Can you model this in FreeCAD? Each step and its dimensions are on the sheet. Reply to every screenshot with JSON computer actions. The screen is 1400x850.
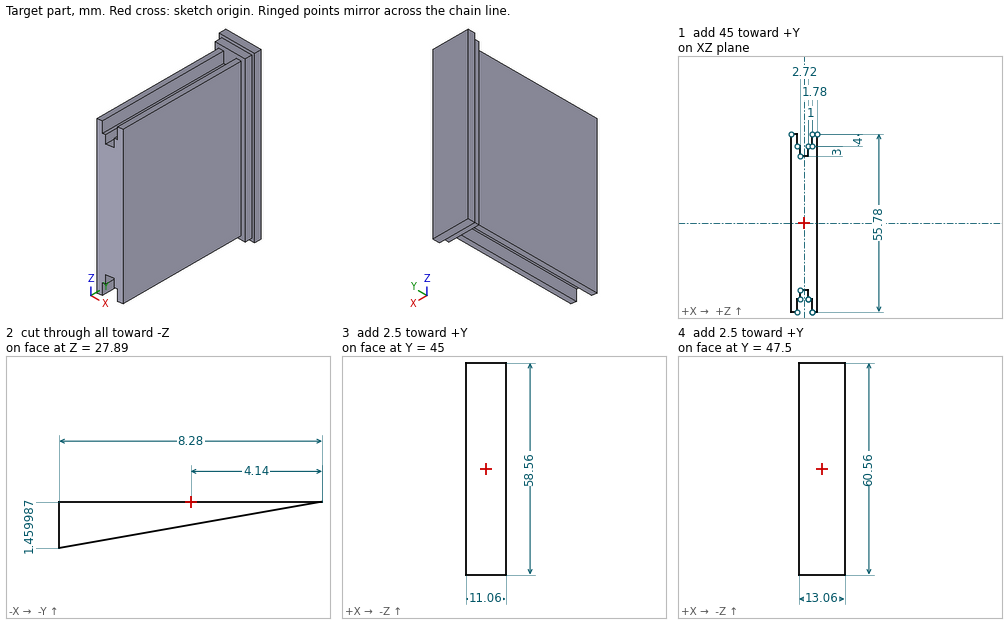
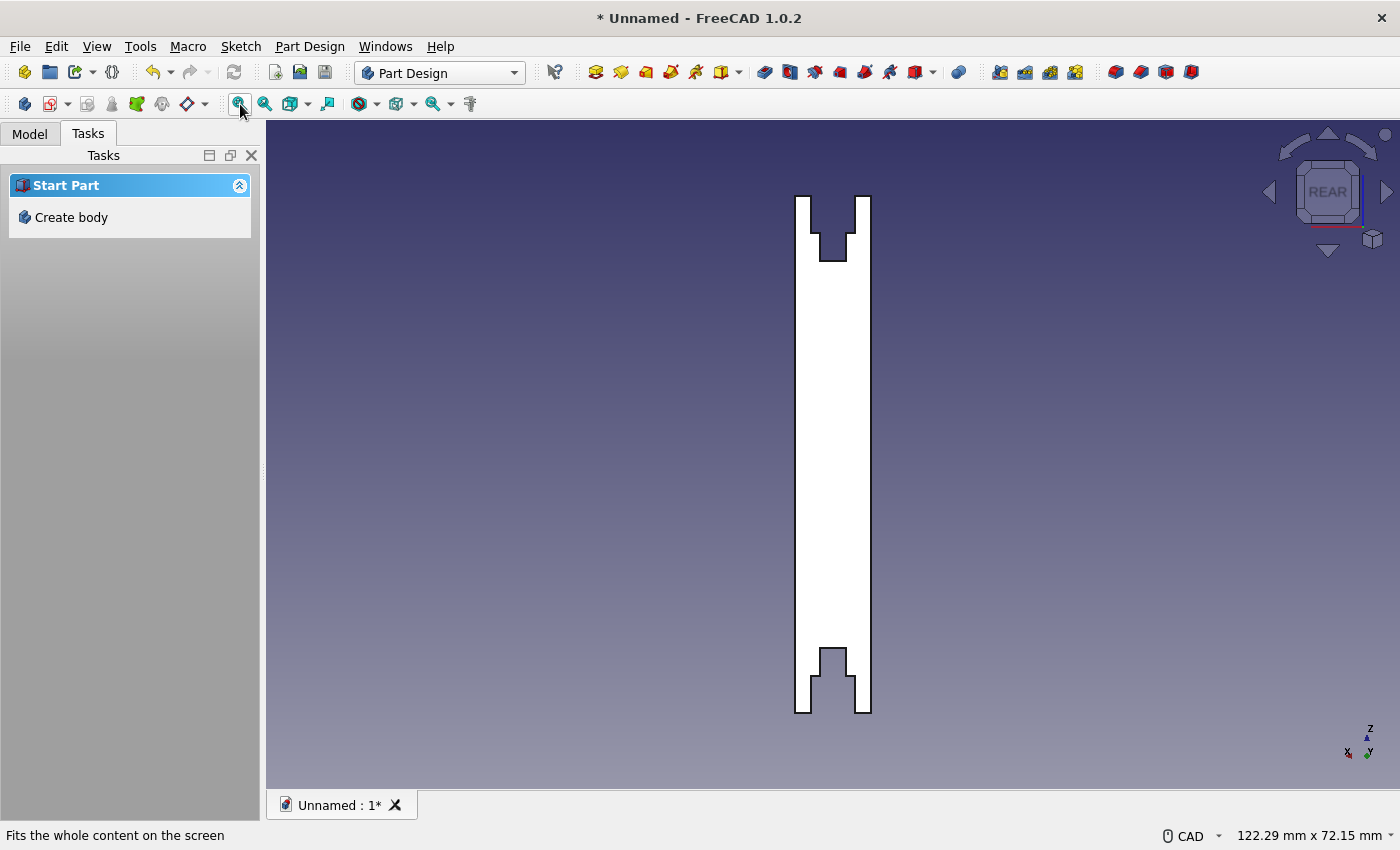
{"action": "left_click", "coordinate": [833, 306]}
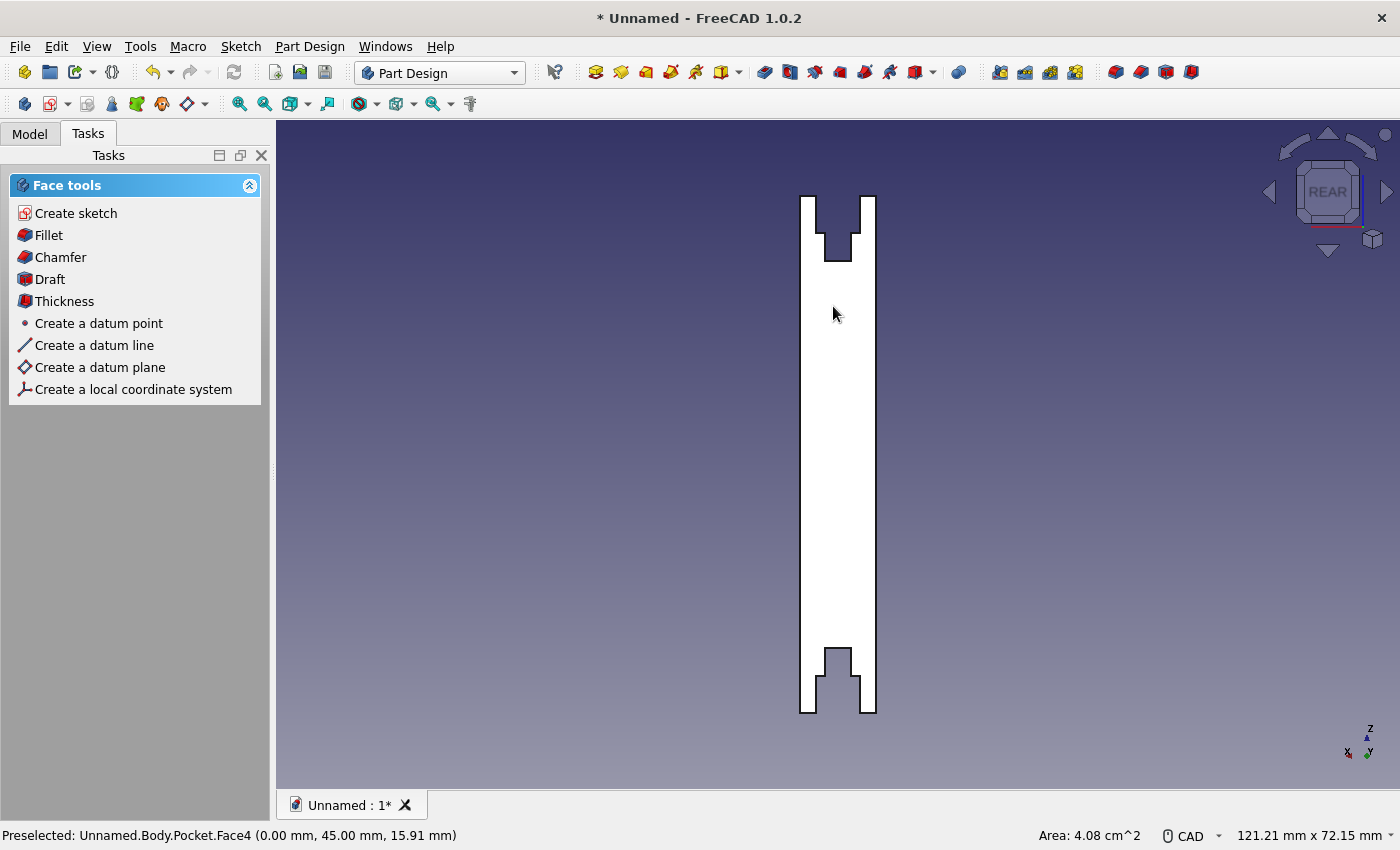
{"action": "left_click", "coordinate": [50, 104]}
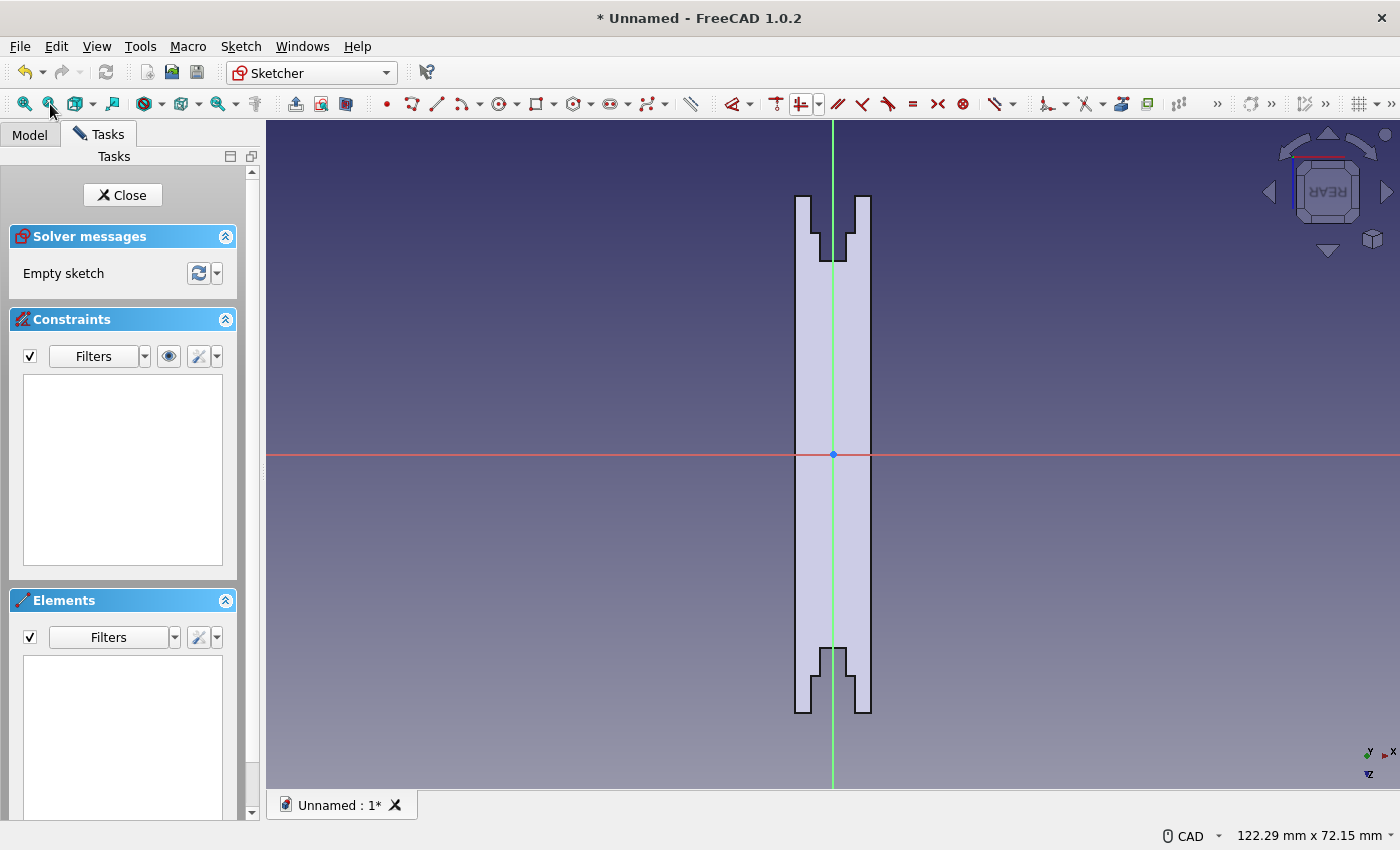
{"action": "key", "text": "g v"}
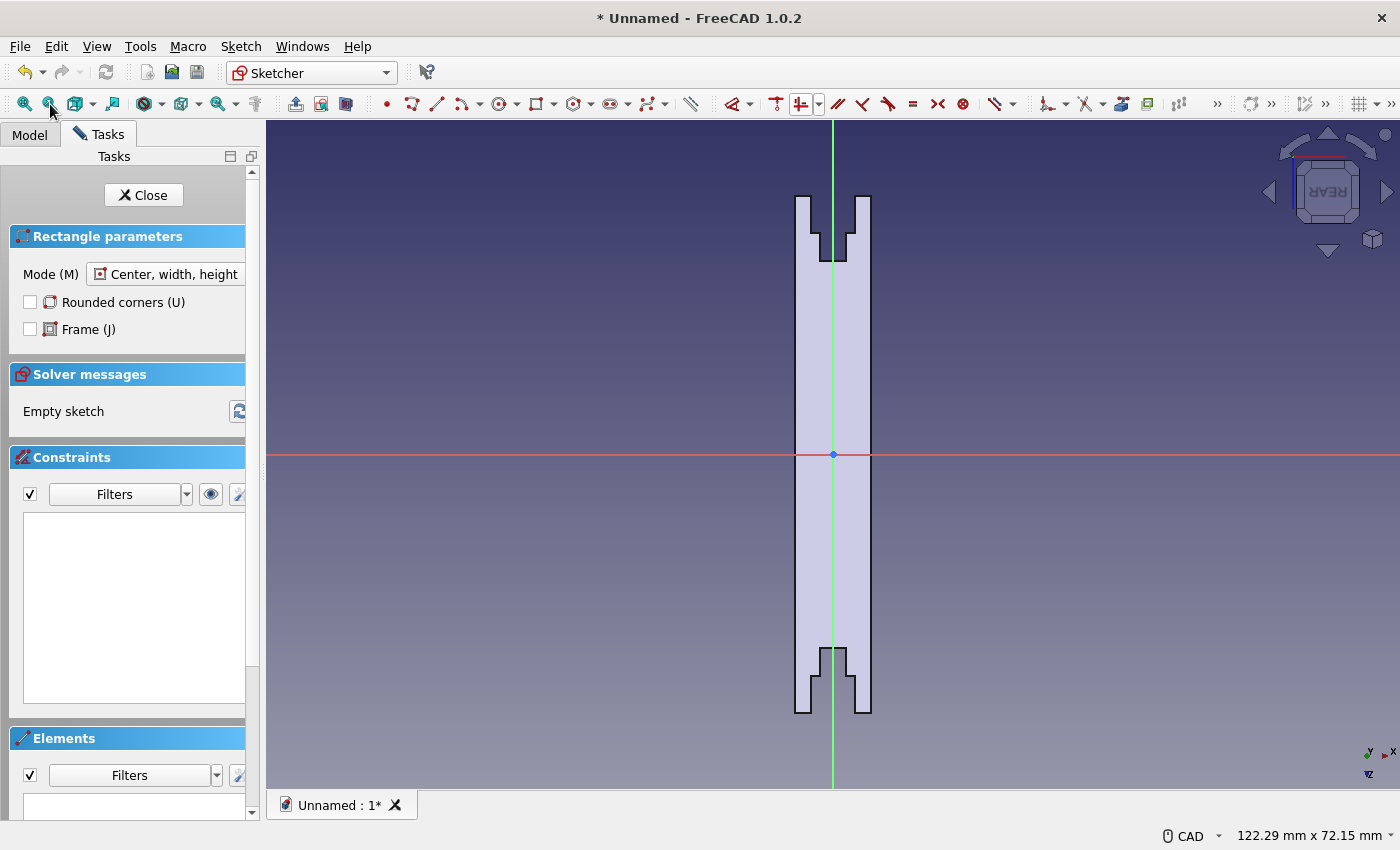
{"action": "left_click", "coordinate": [833, 454]}
{"action": "left_click", "coordinate": [884, 183]}
{"action": "key", "text": "Escape"}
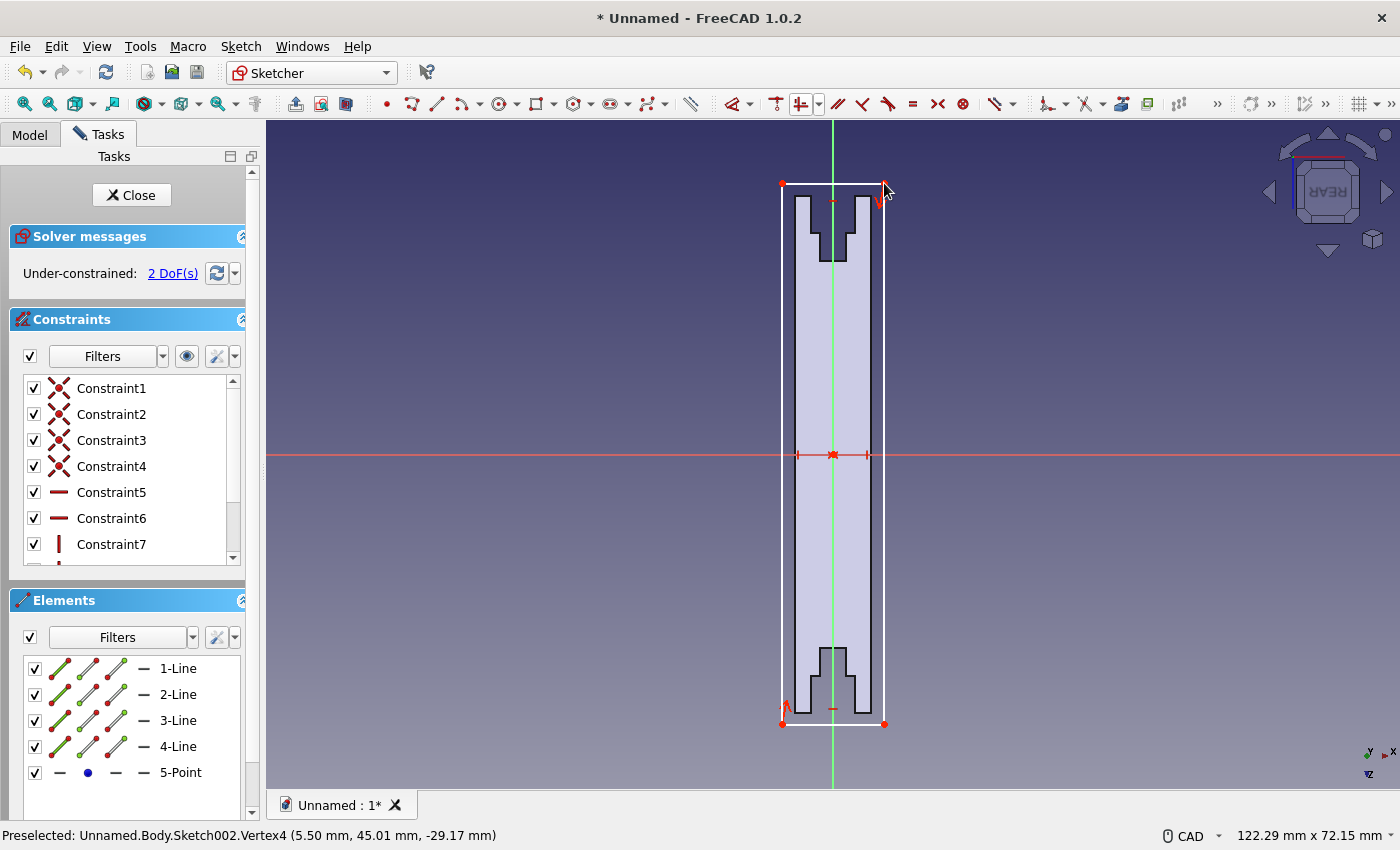
{"action": "left_click", "coordinate": [732, 104]}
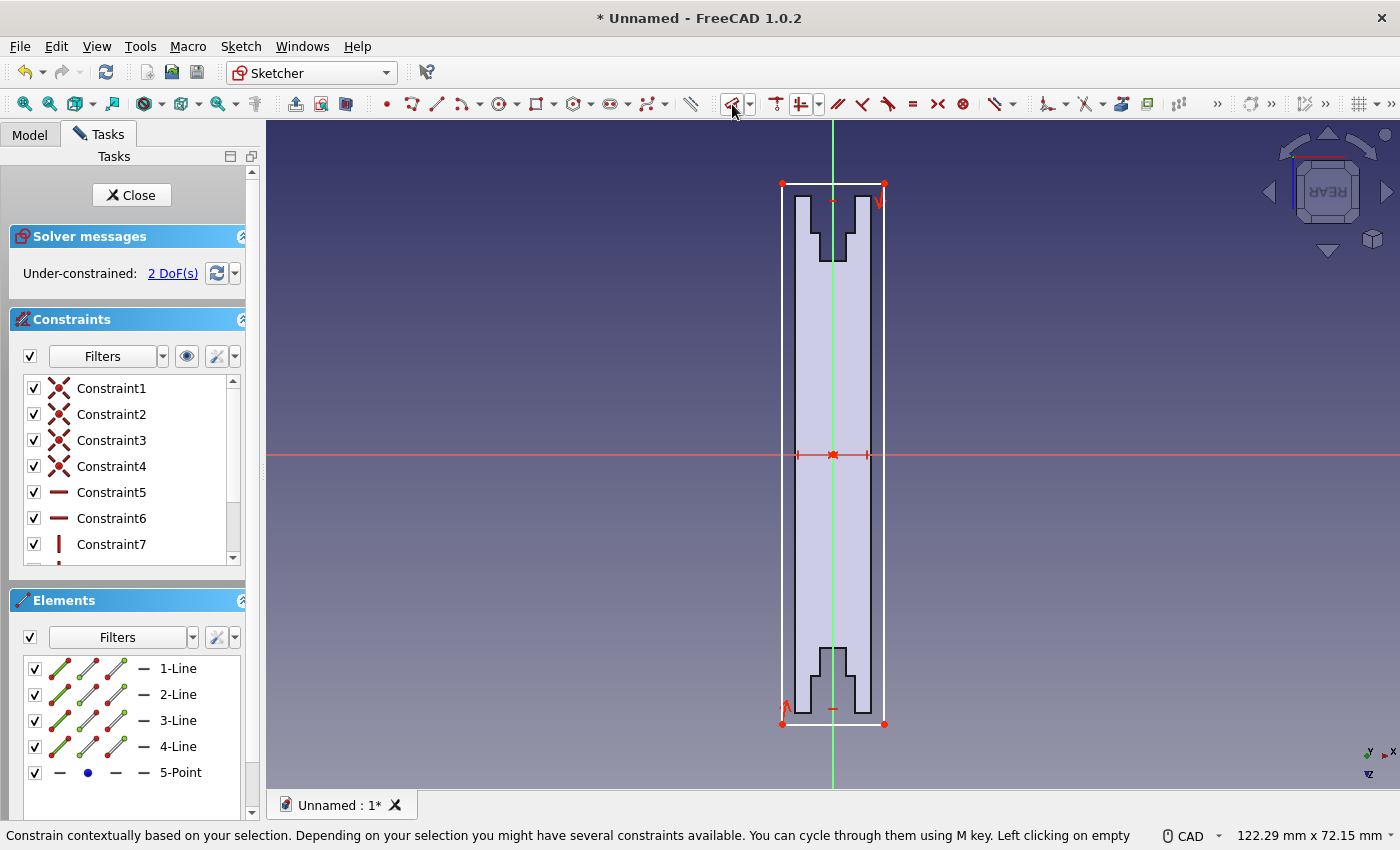
{"action": "left_click", "coordinate": [813, 725]}
{"action": "left_click", "coordinate": [810, 759]}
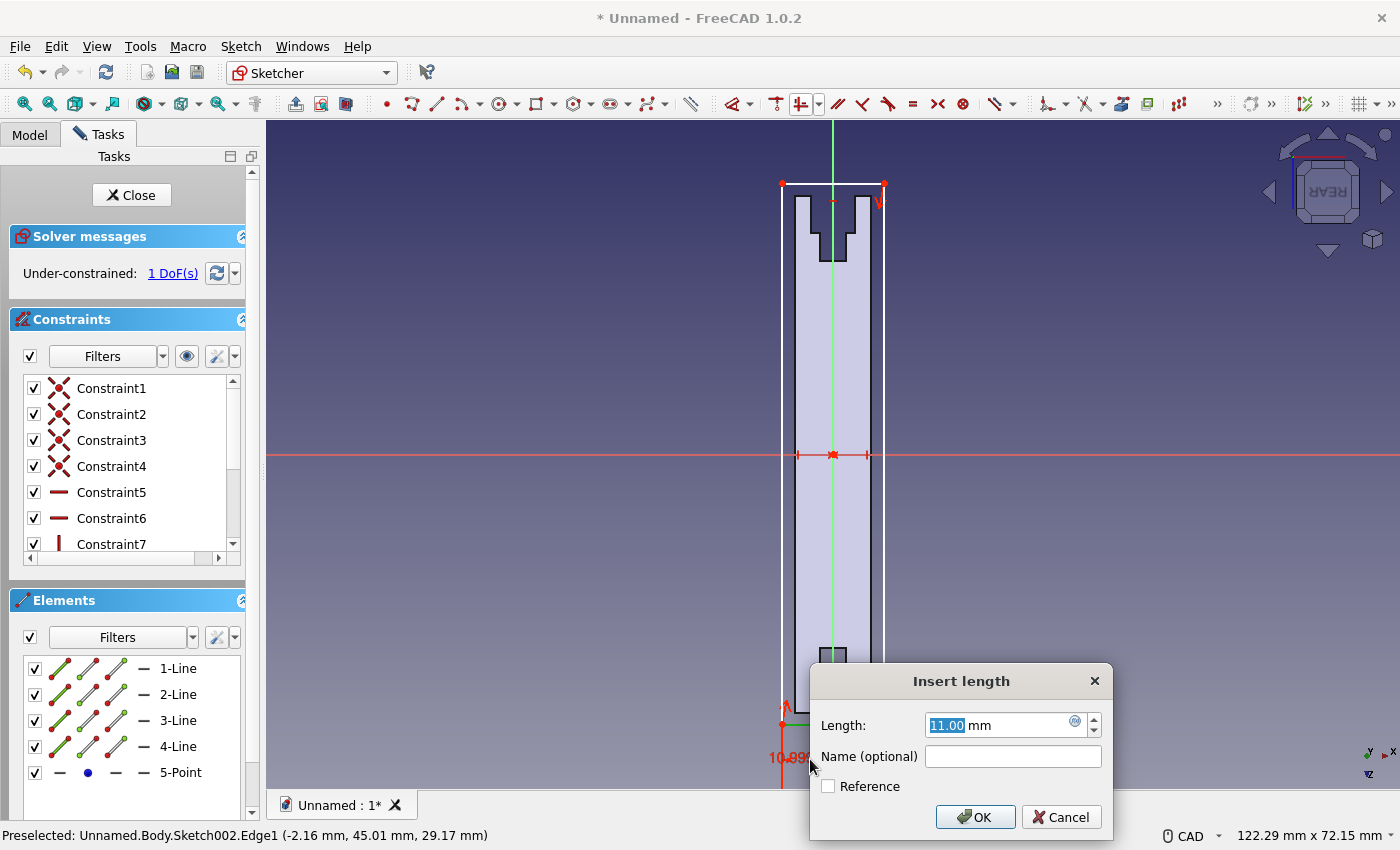
{"action": "type", "text": "11.06"}
{"action": "key", "text": "Return"}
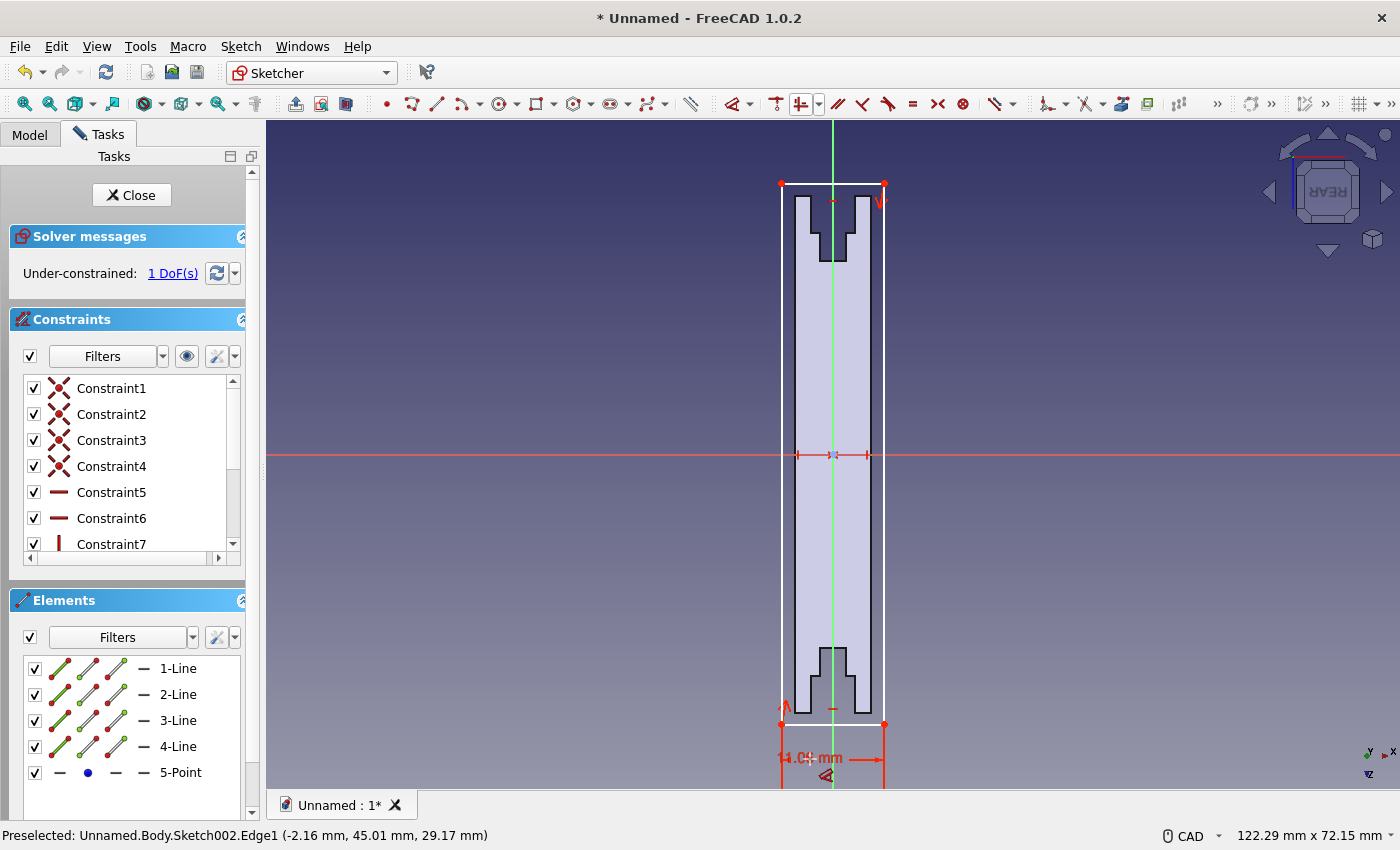
{"action": "left_click", "coordinate": [884, 563]}
{"action": "left_click", "coordinate": [918, 330]}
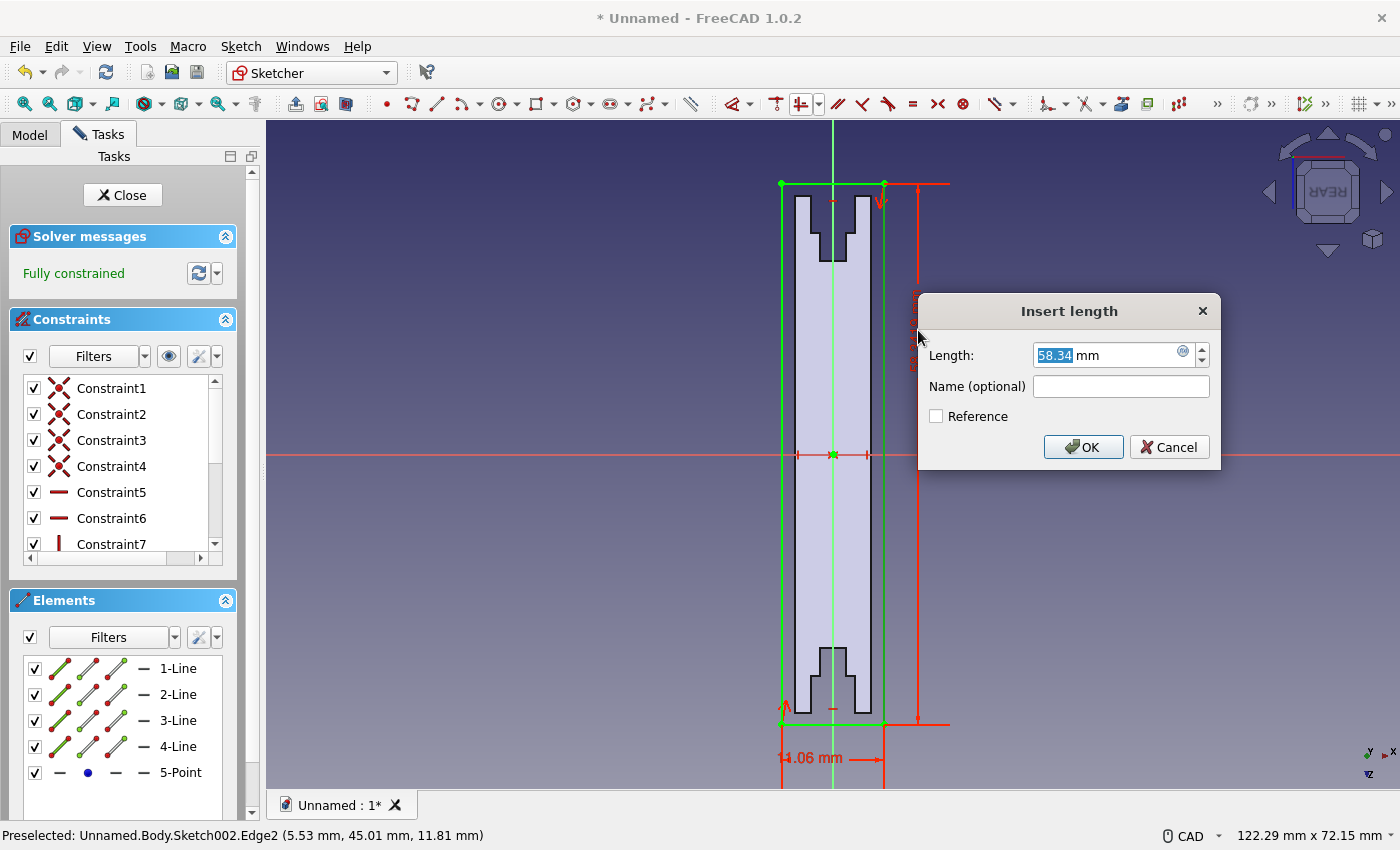
{"action": "type", "text": "58.56"}
{"action": "key", "text": "Return"}
{"action": "key", "text": "Escape"}